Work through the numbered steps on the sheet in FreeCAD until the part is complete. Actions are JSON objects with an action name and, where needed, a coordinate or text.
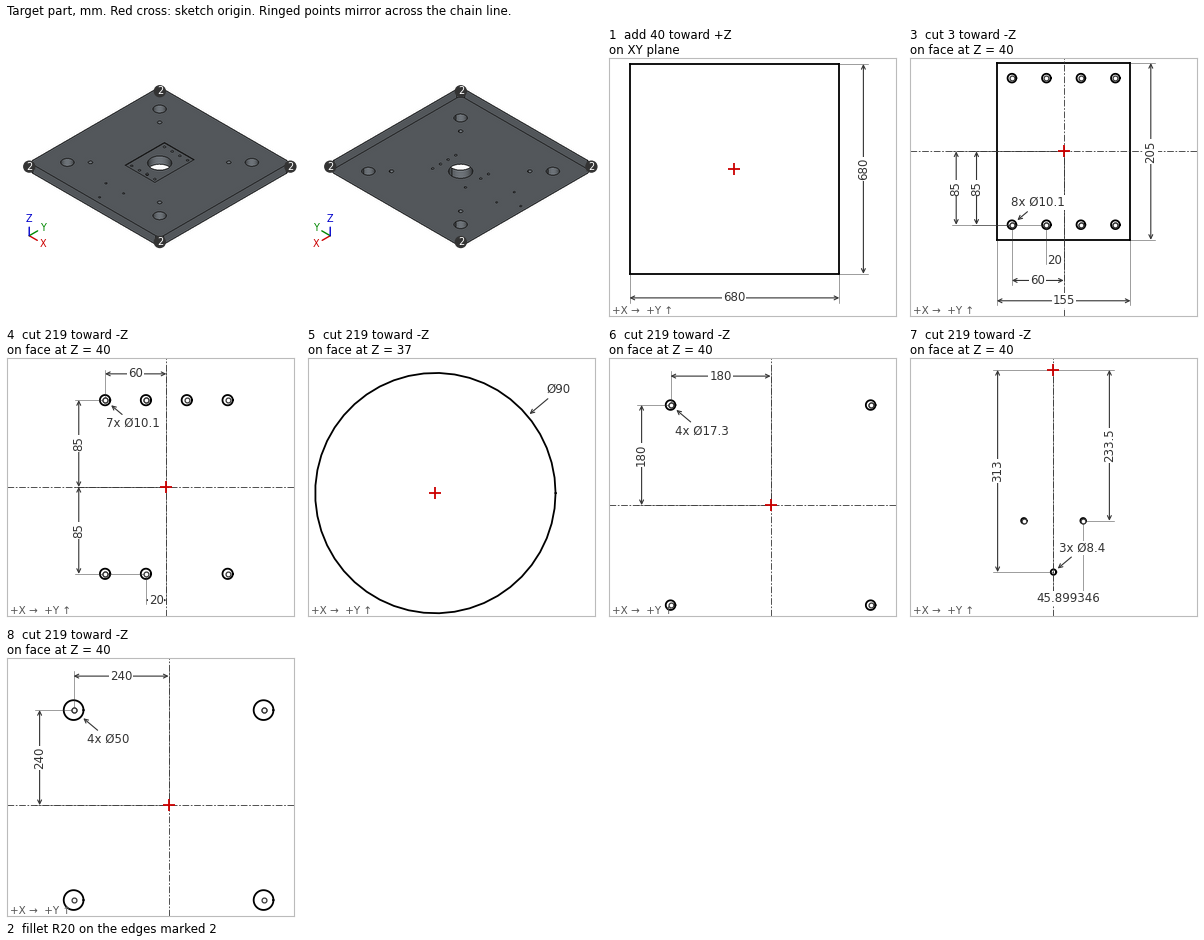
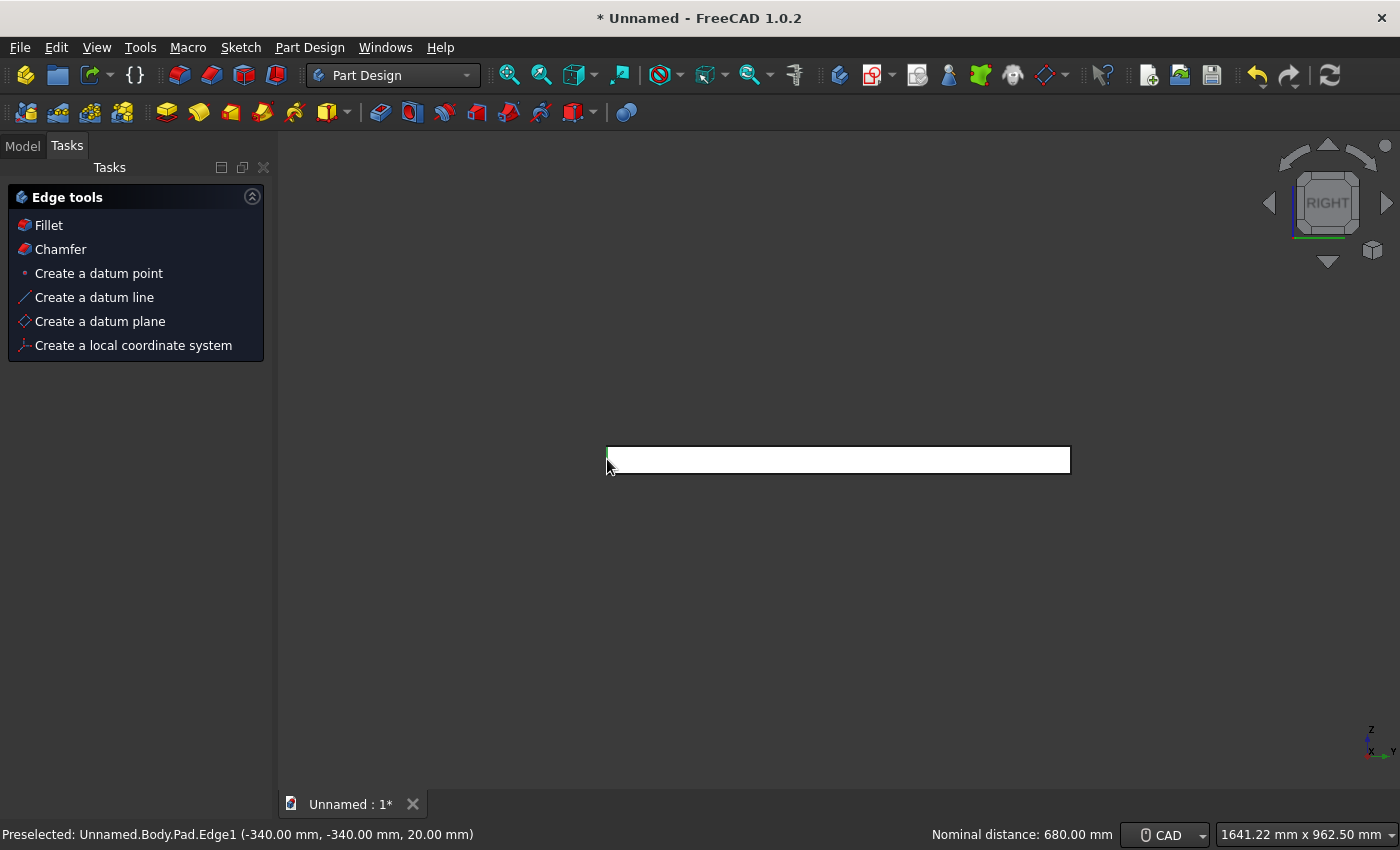
{"action": "left_click", "coordinate": [510, 76]}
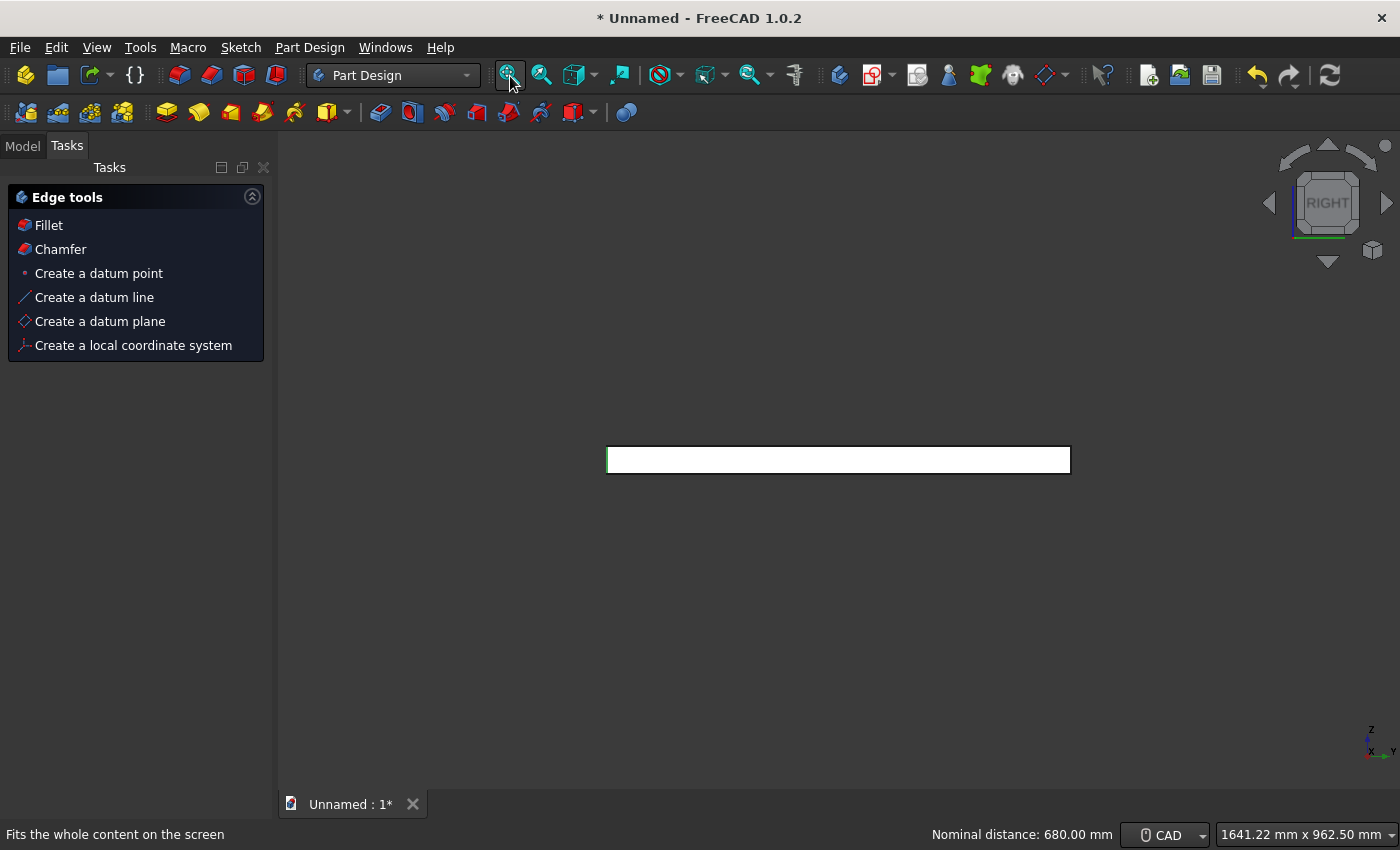
{"action": "left_click", "coordinate": [1071, 459], "text": "ctrl"}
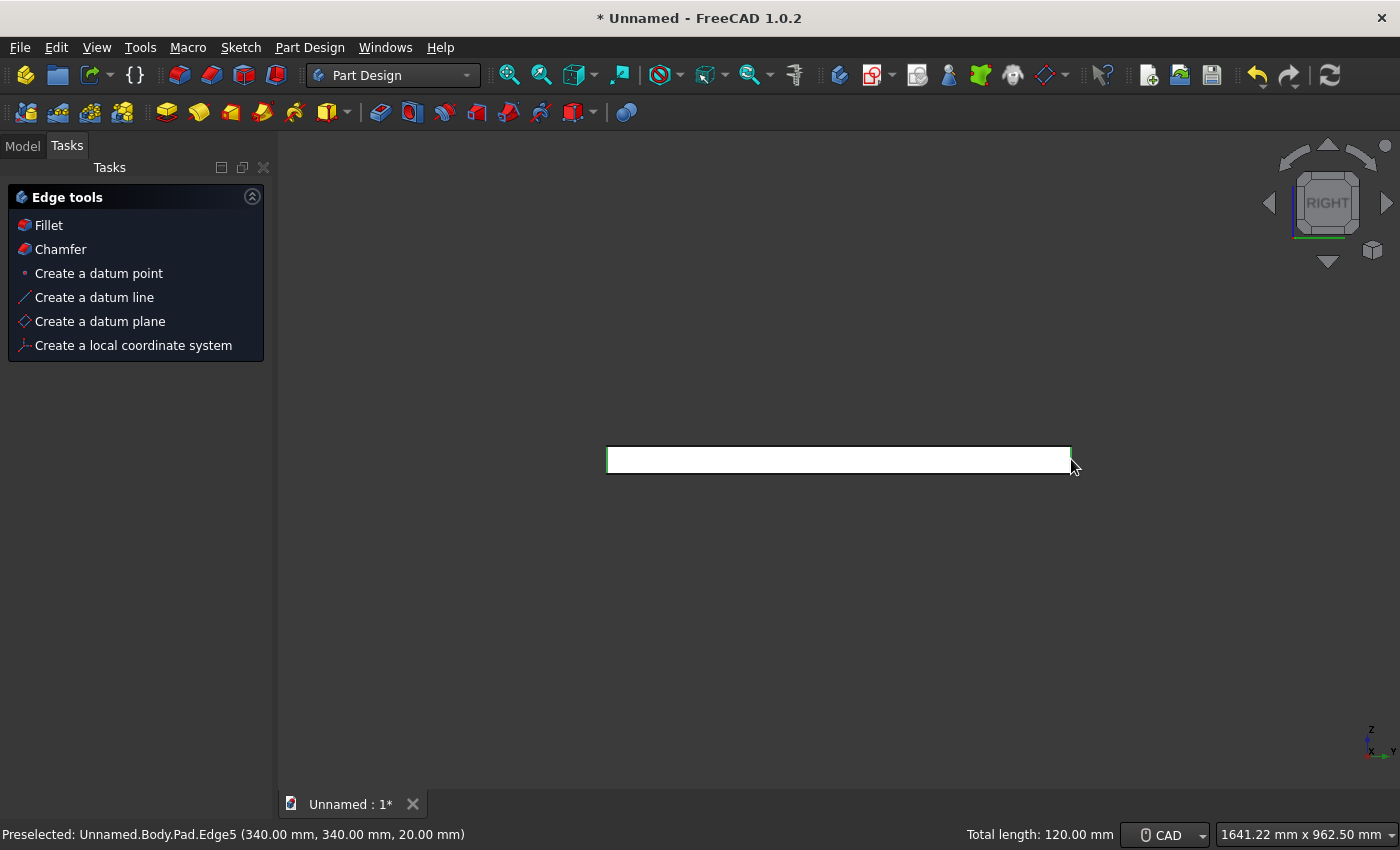
{"action": "key", "text": "5"}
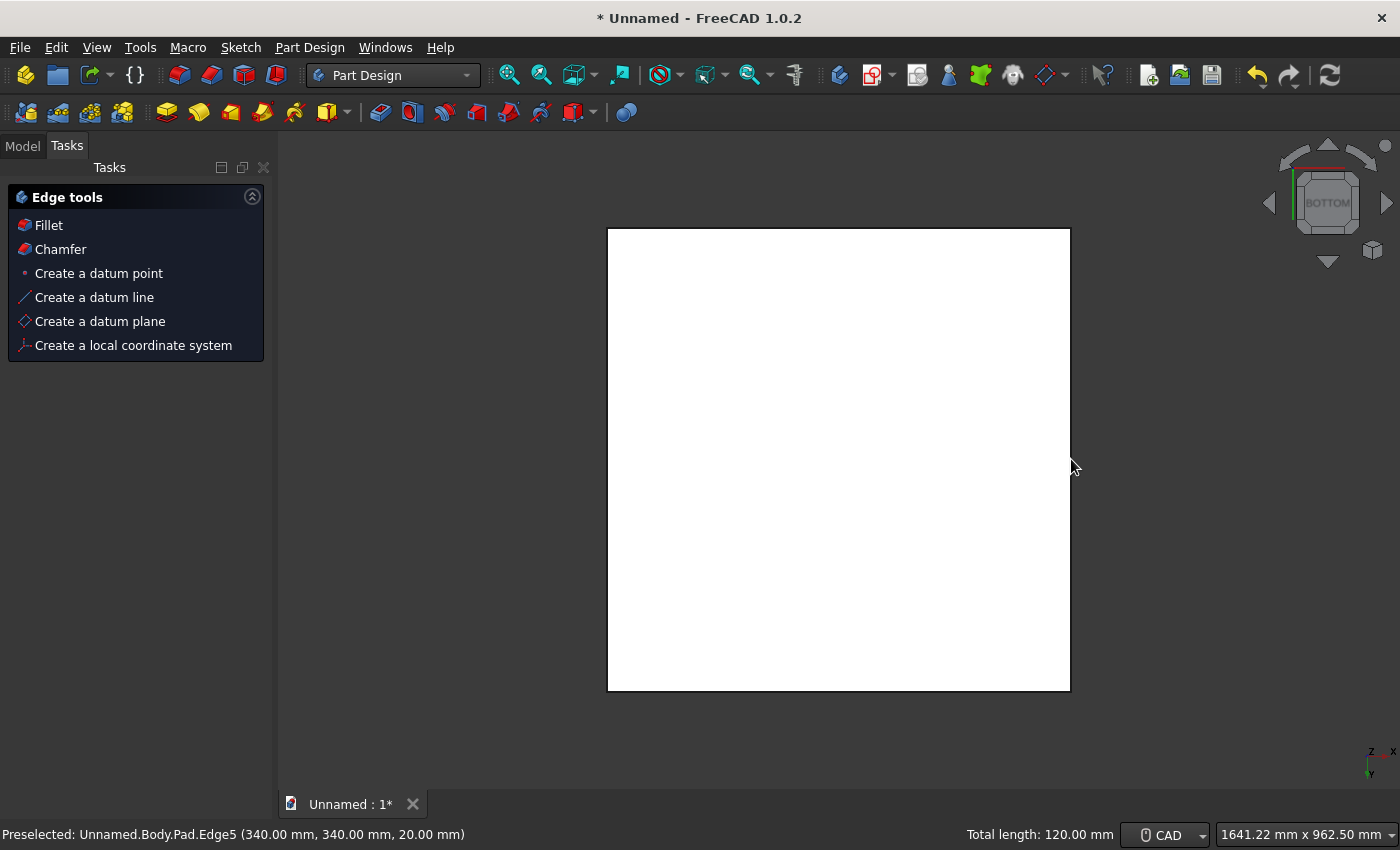
{"action": "key", "text": "4"}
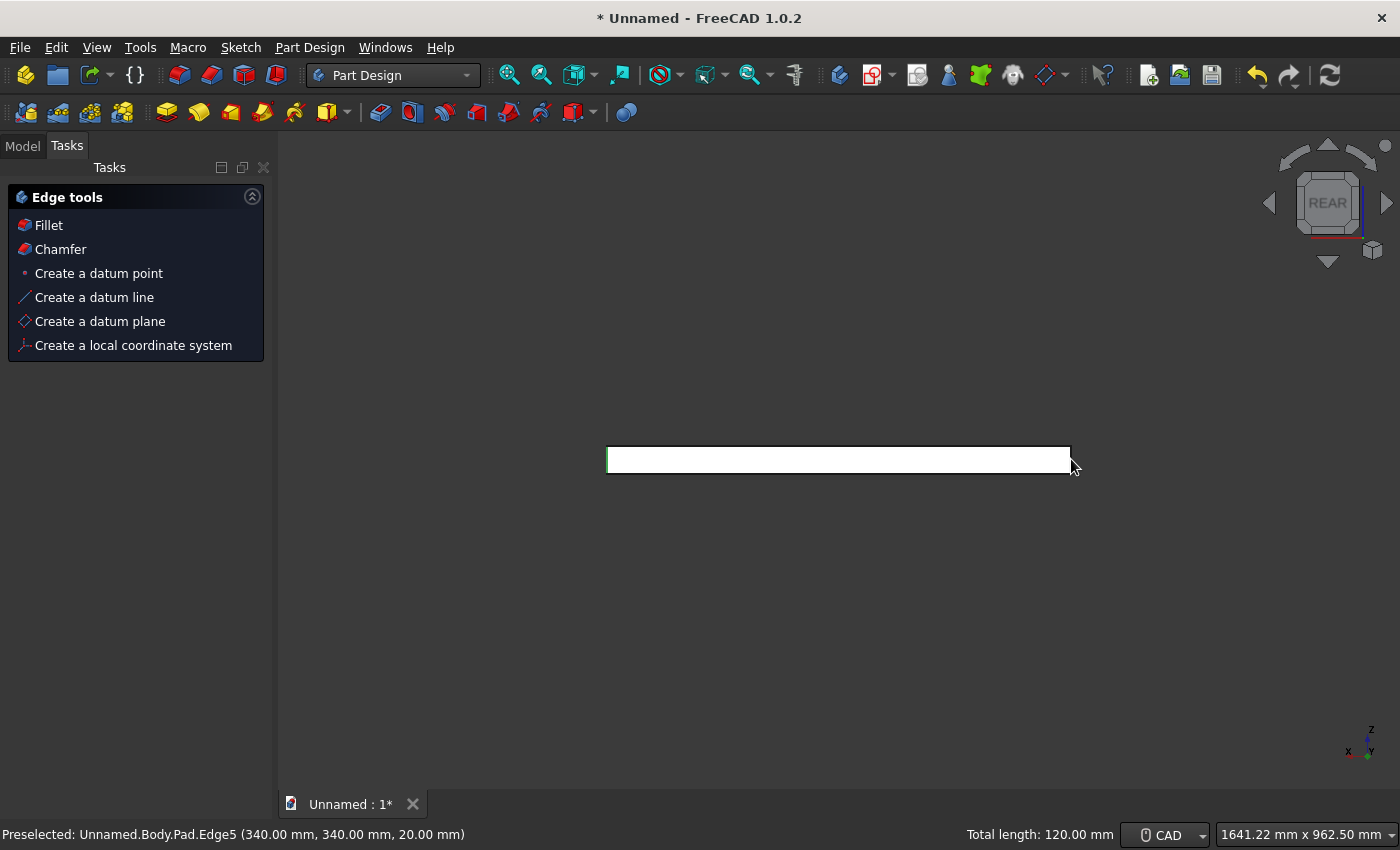
{"action": "left_click", "coordinate": [510, 76]}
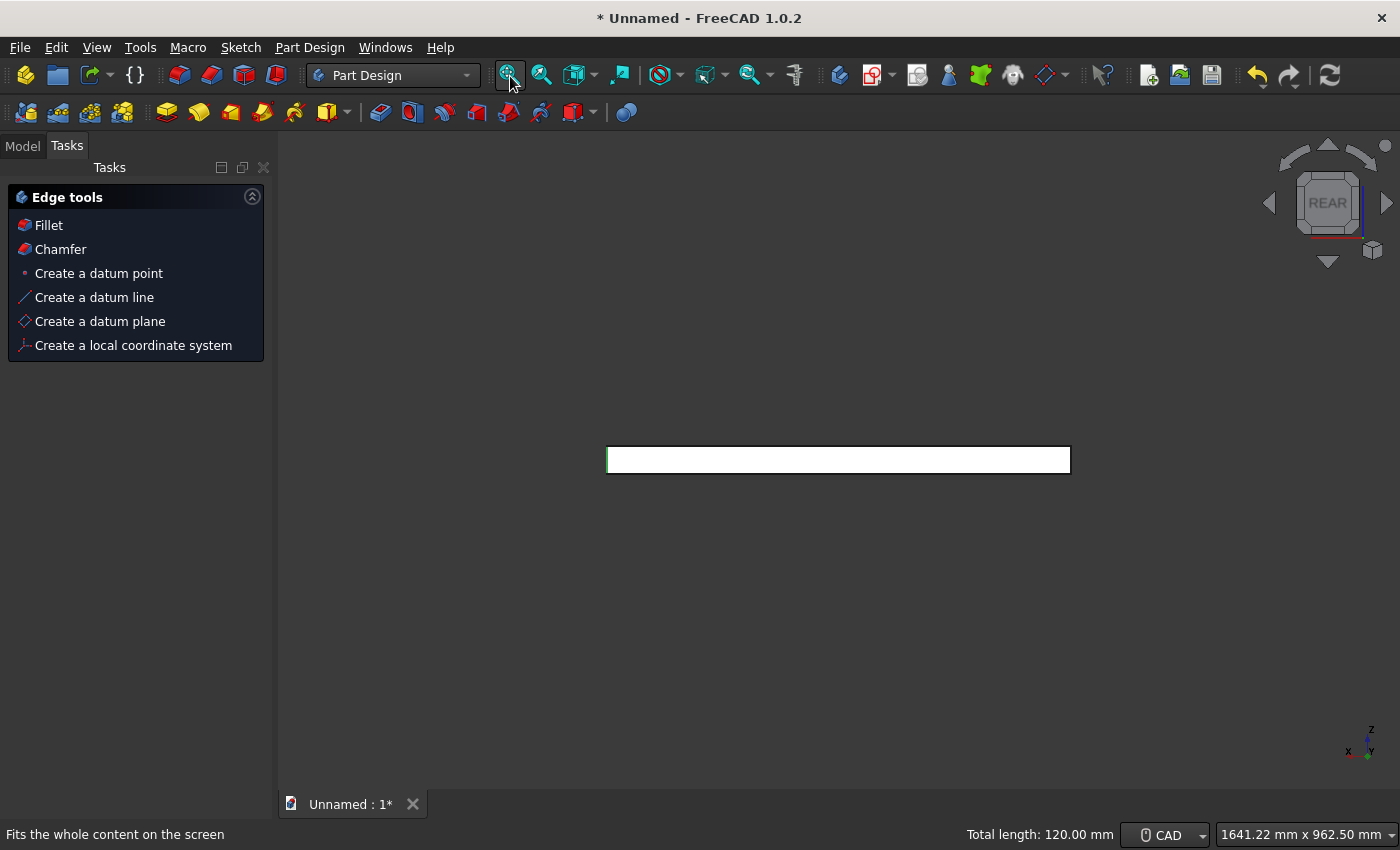
{"action": "left_click", "coordinate": [1071, 459], "text": "ctrl"}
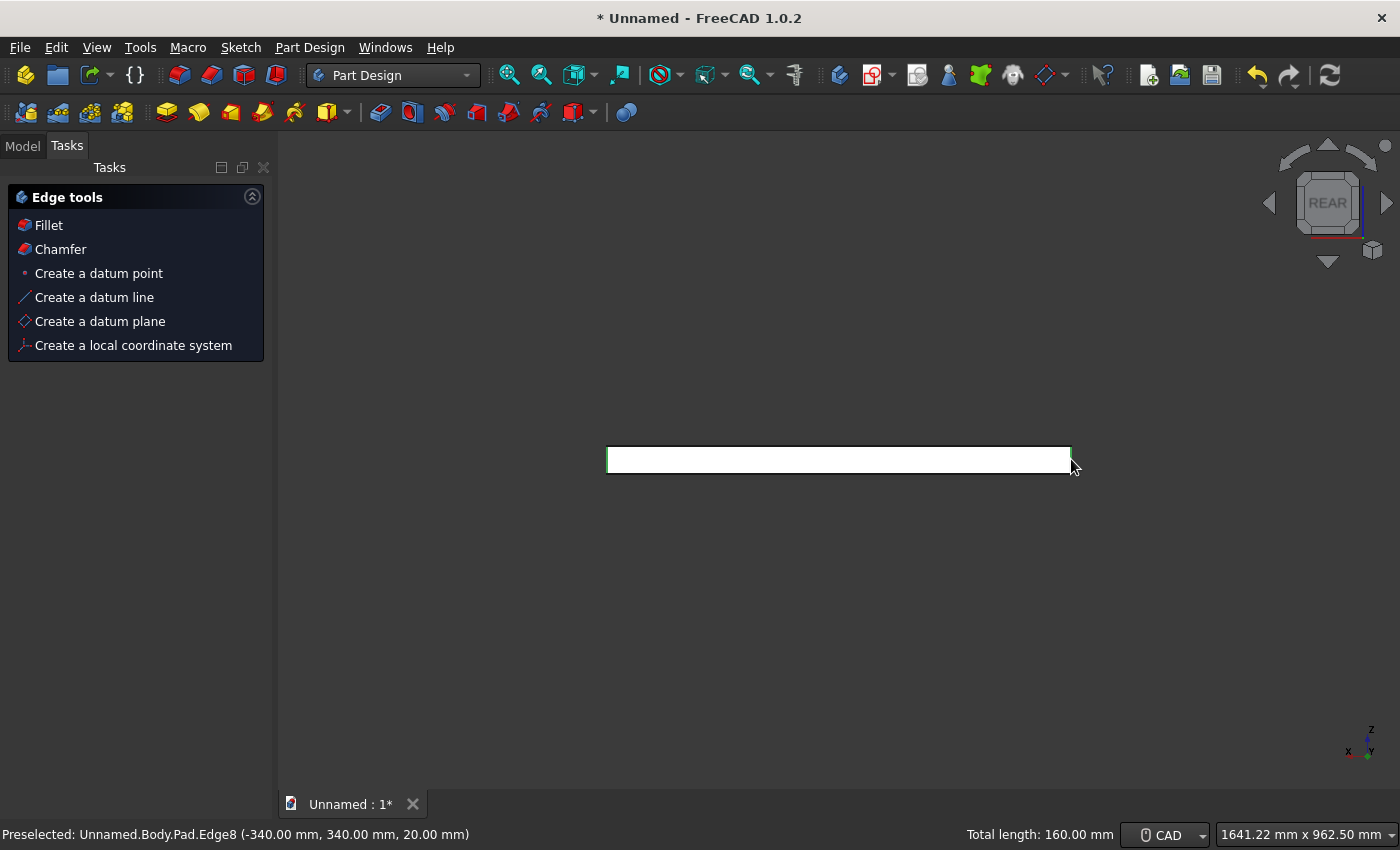
{"action": "left_click", "coordinate": [180, 76]}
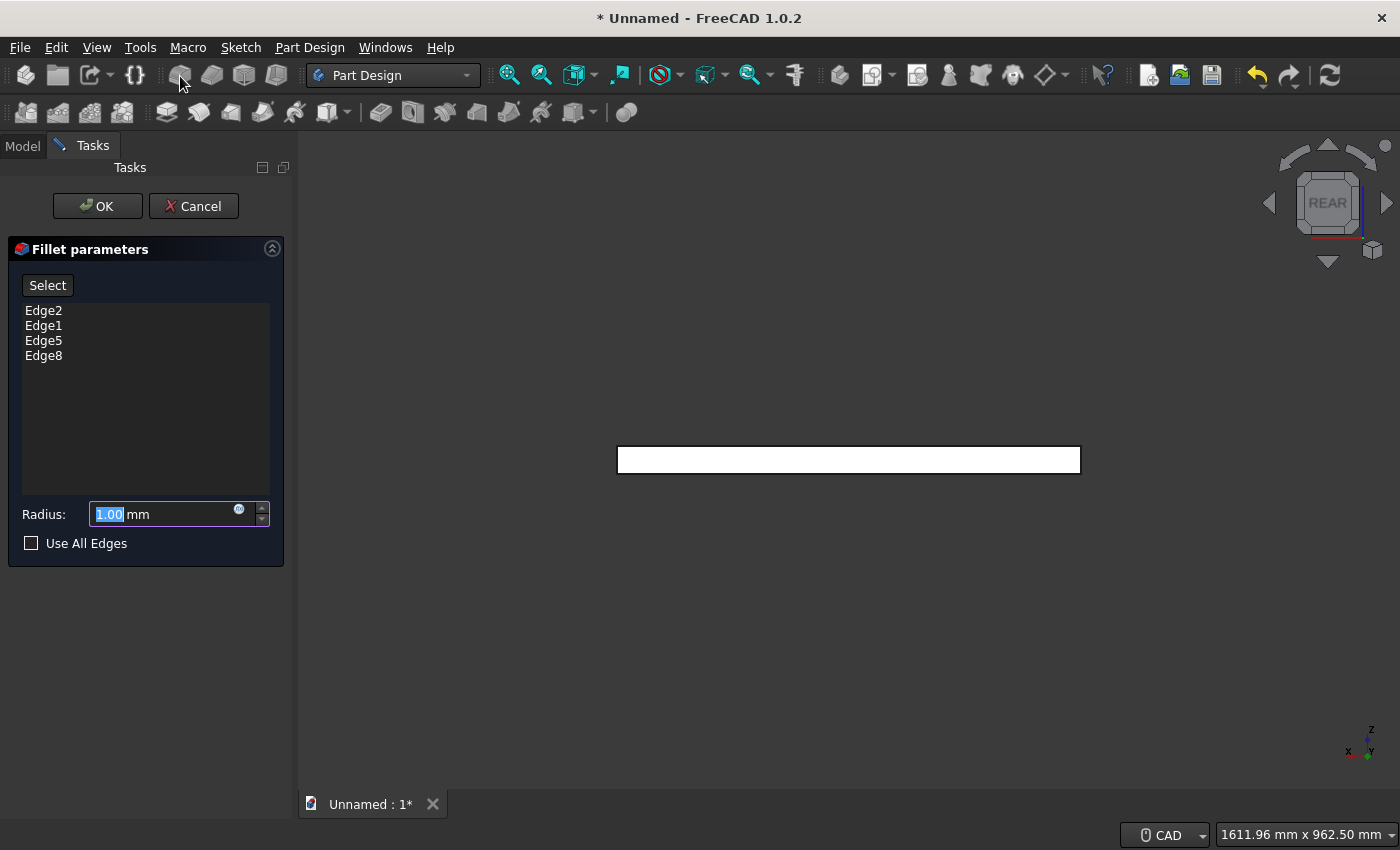
{"action": "type", "text": "20"}
{"action": "key", "text": "Tab"}